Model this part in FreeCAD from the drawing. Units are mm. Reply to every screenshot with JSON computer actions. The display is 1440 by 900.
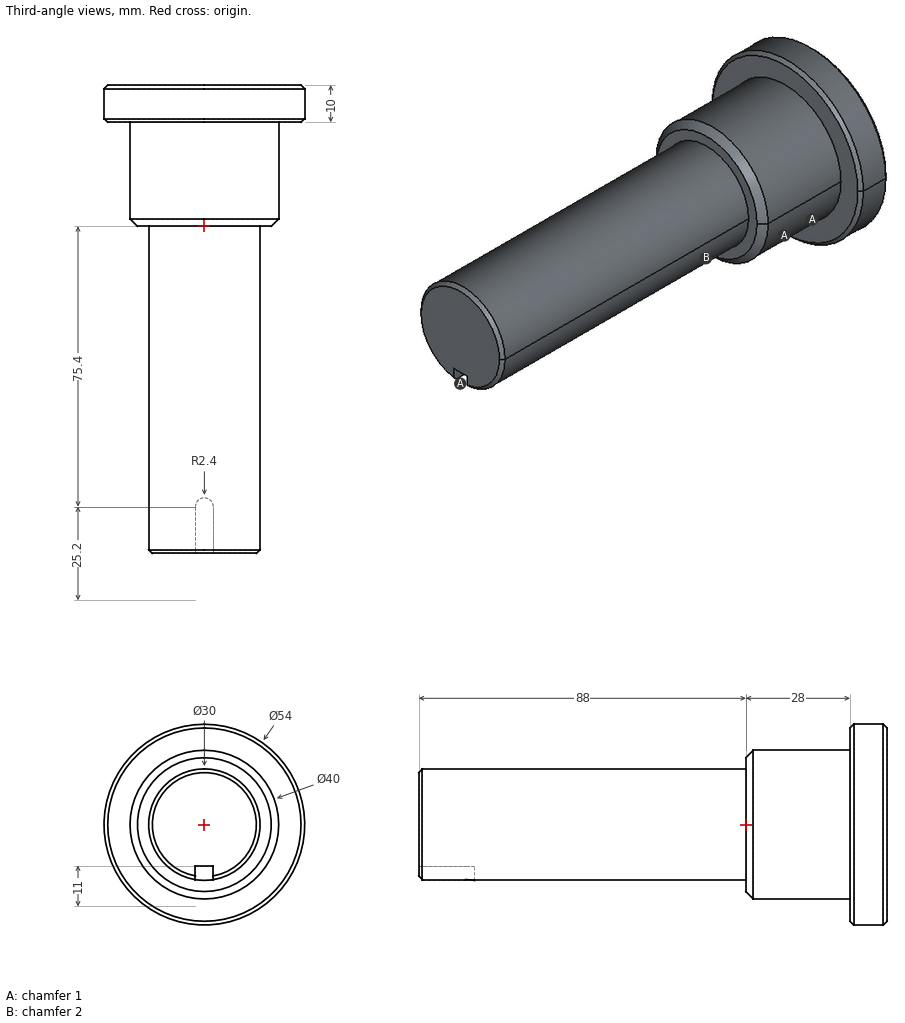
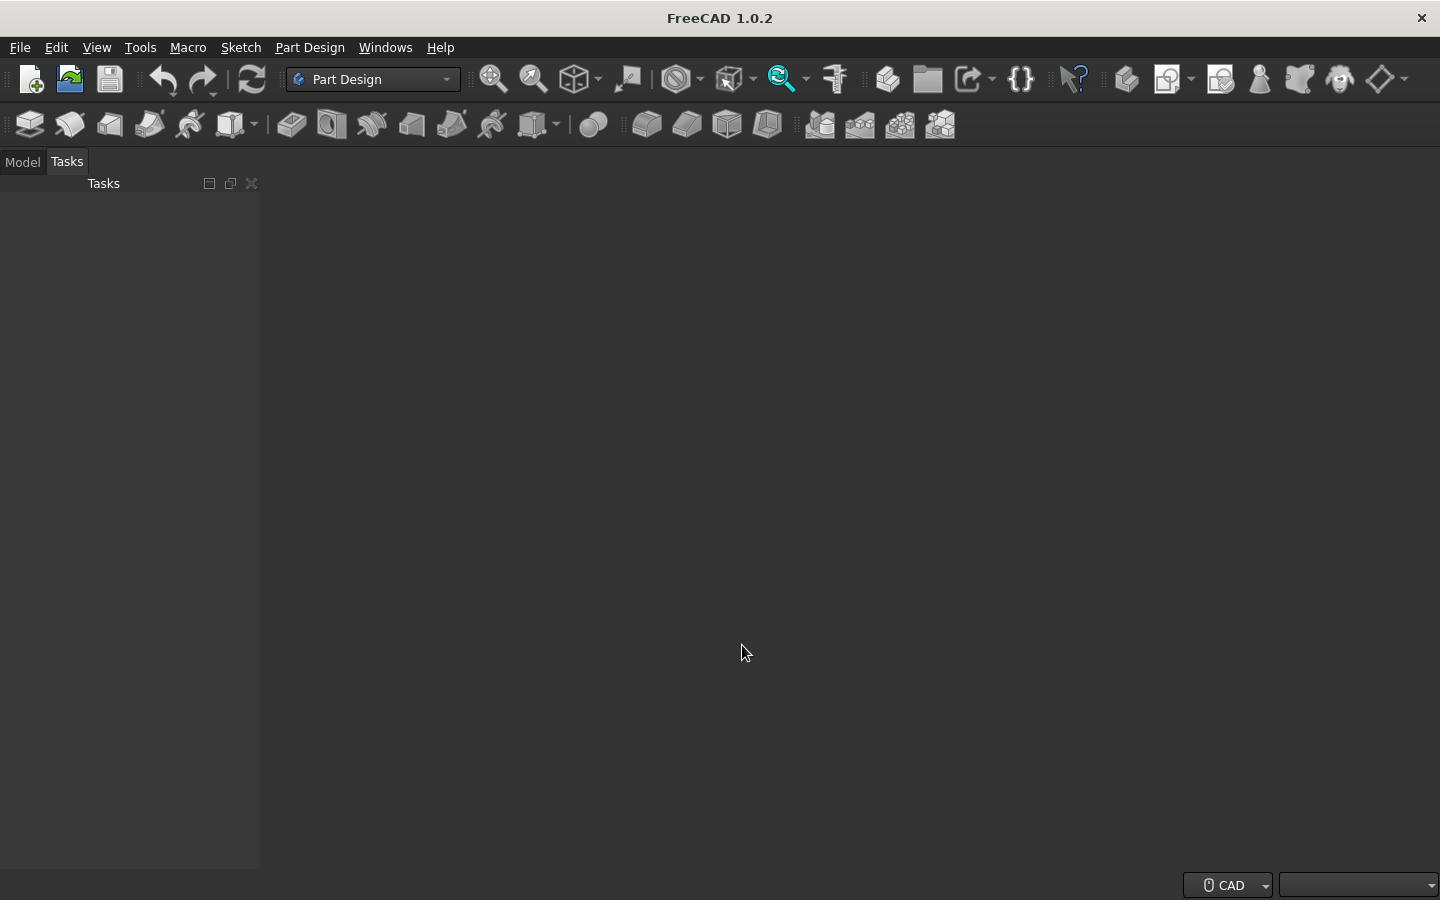
{"action": "left_click", "coordinate": [30, 80]}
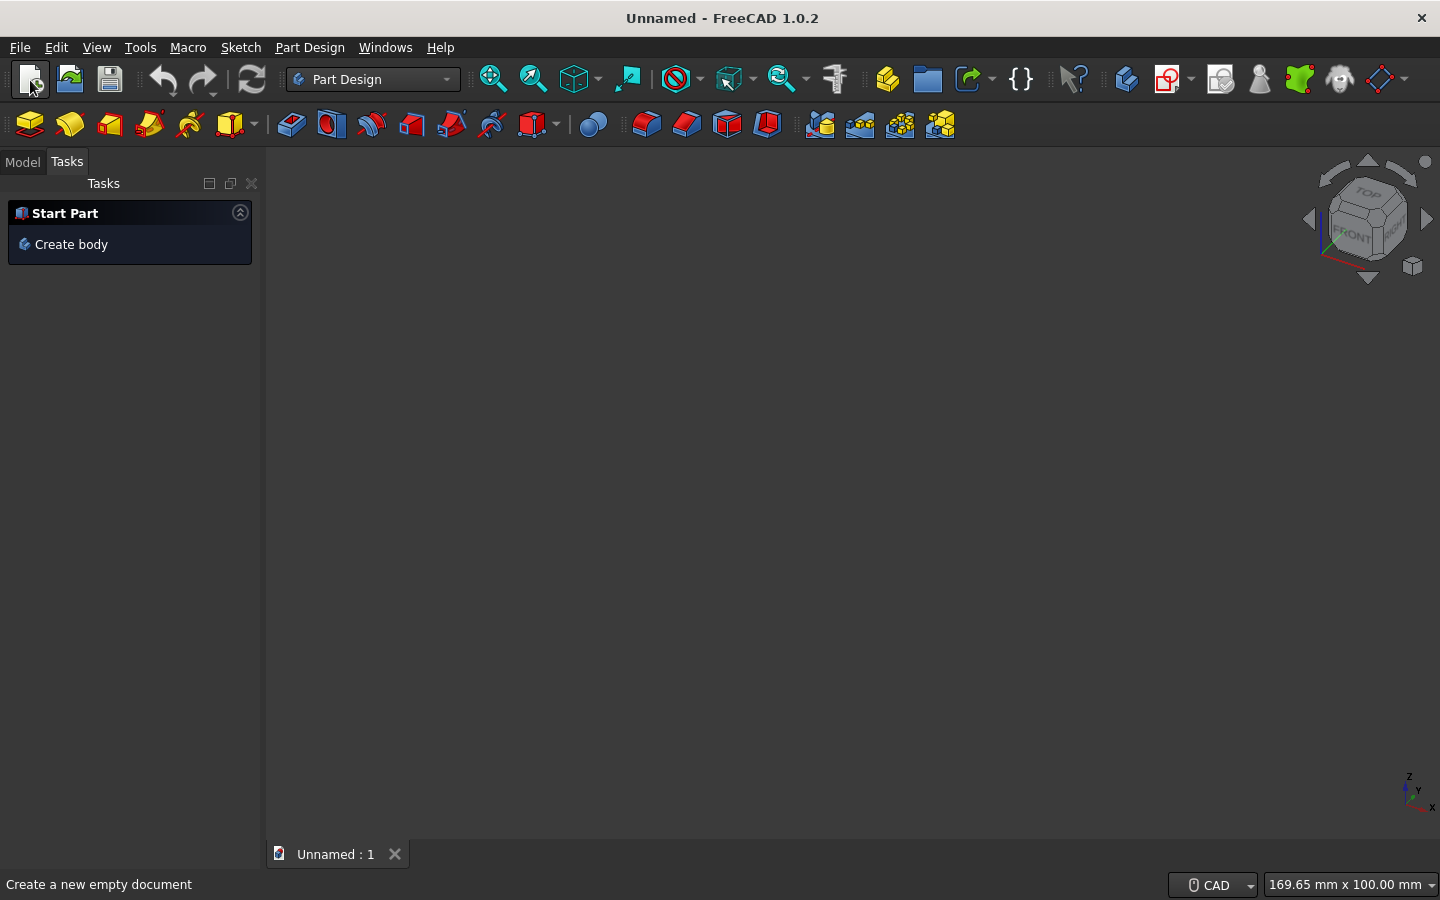
{"action": "left_click", "coordinate": [1168, 80]}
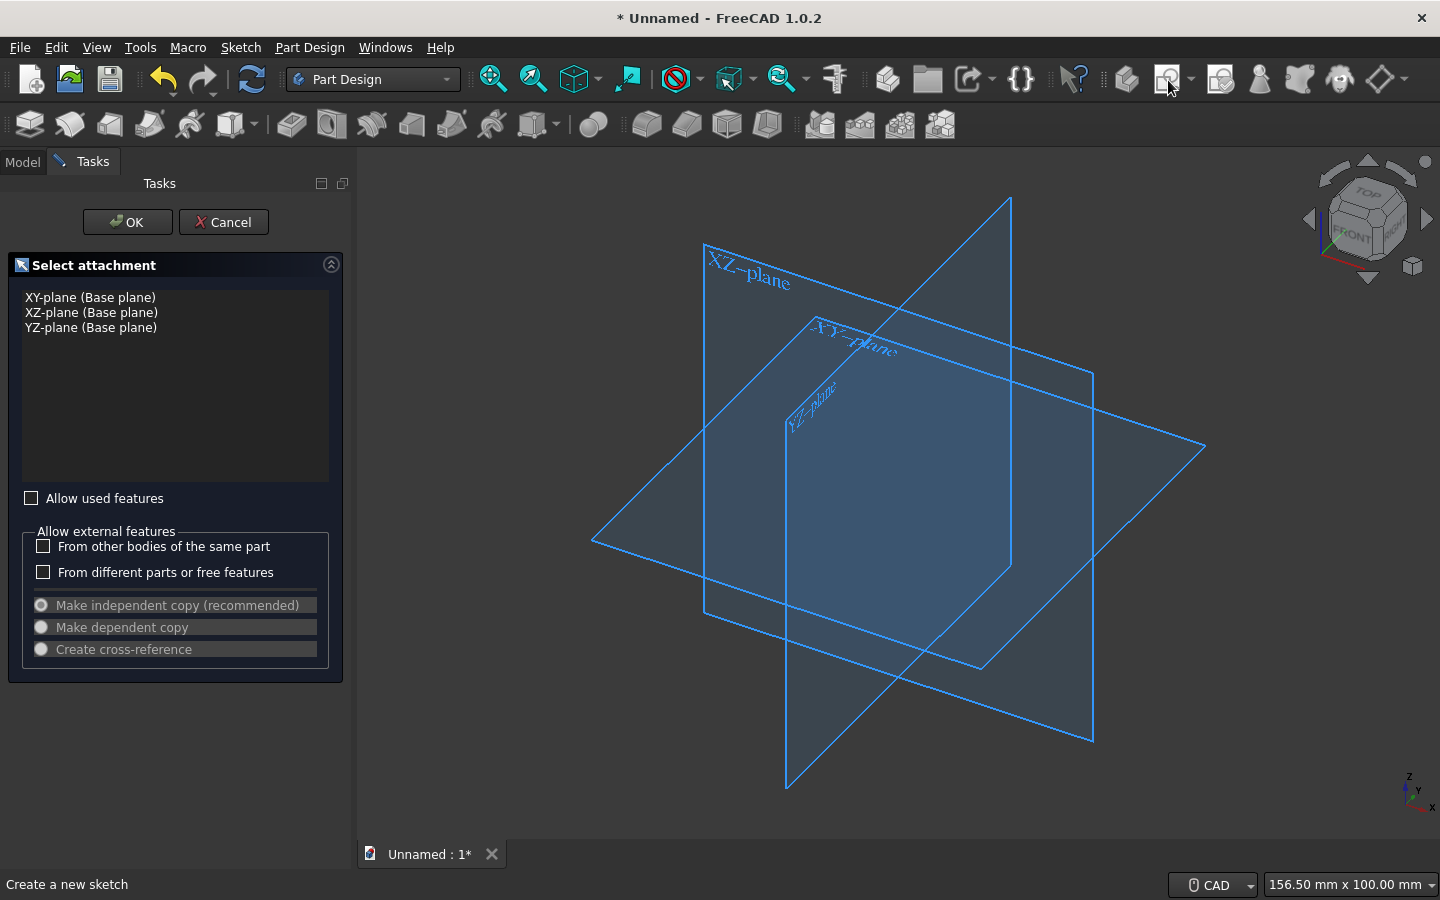
{"action": "left_click", "coordinate": [82, 312]}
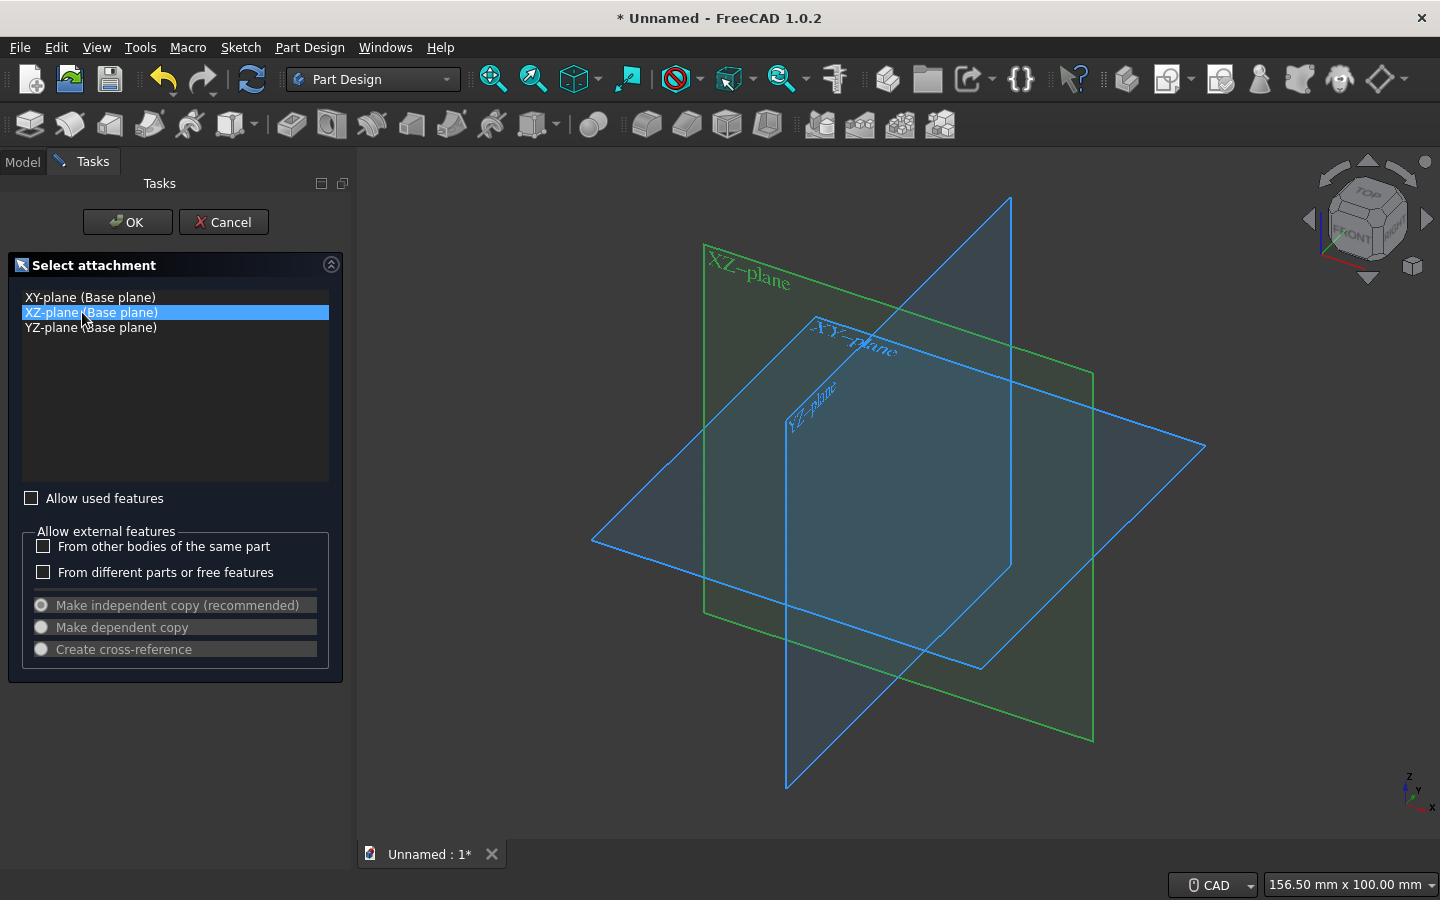
{"action": "left_click", "coordinate": [128, 222]}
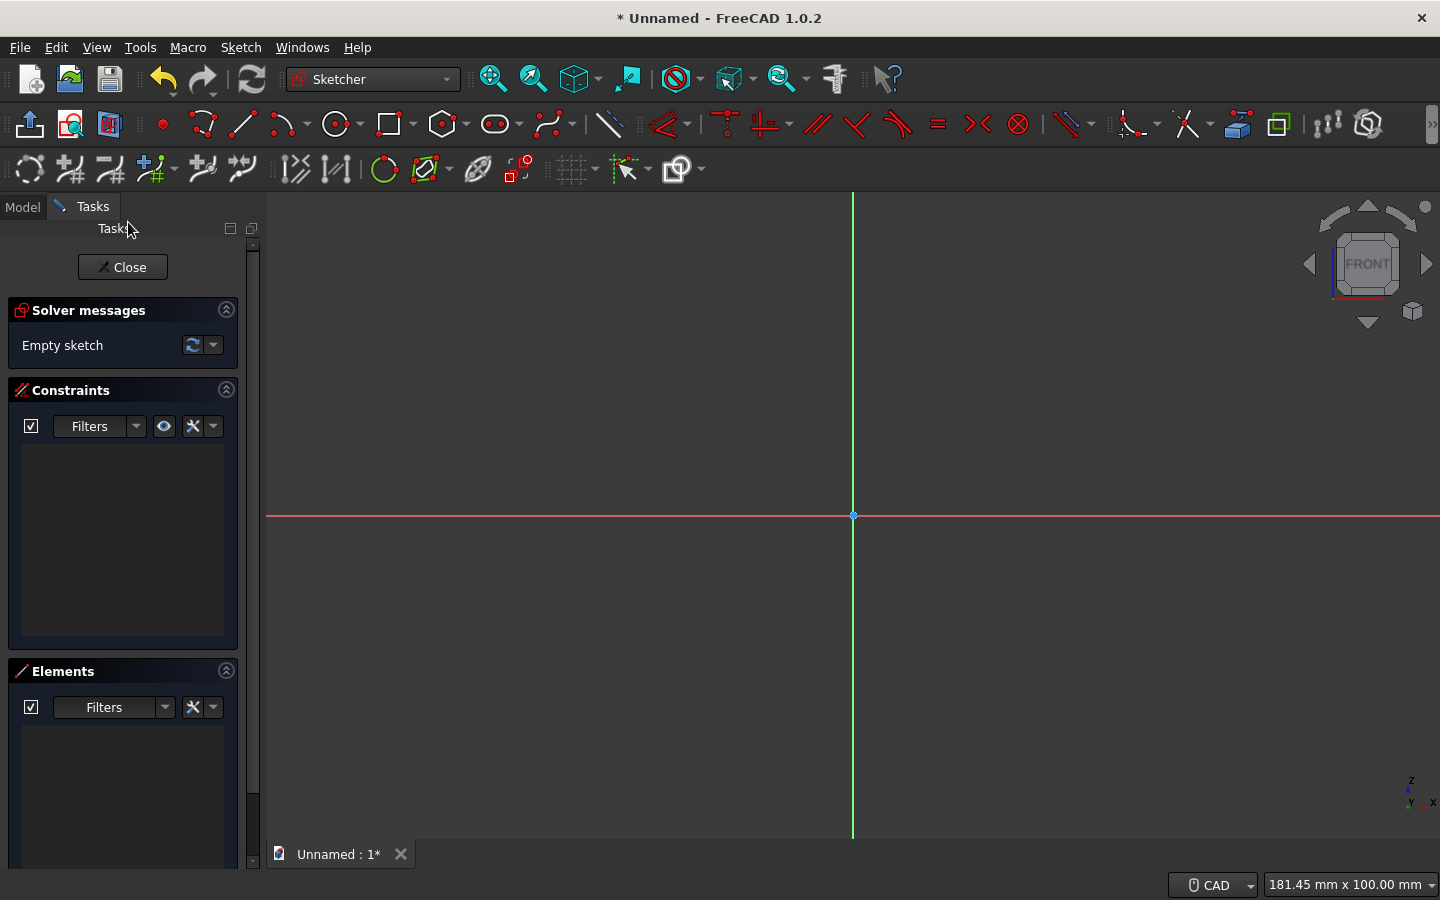
{"action": "scroll", "coordinate": [992, 516], "scroll_direction": "up", "scroll_amount": 2}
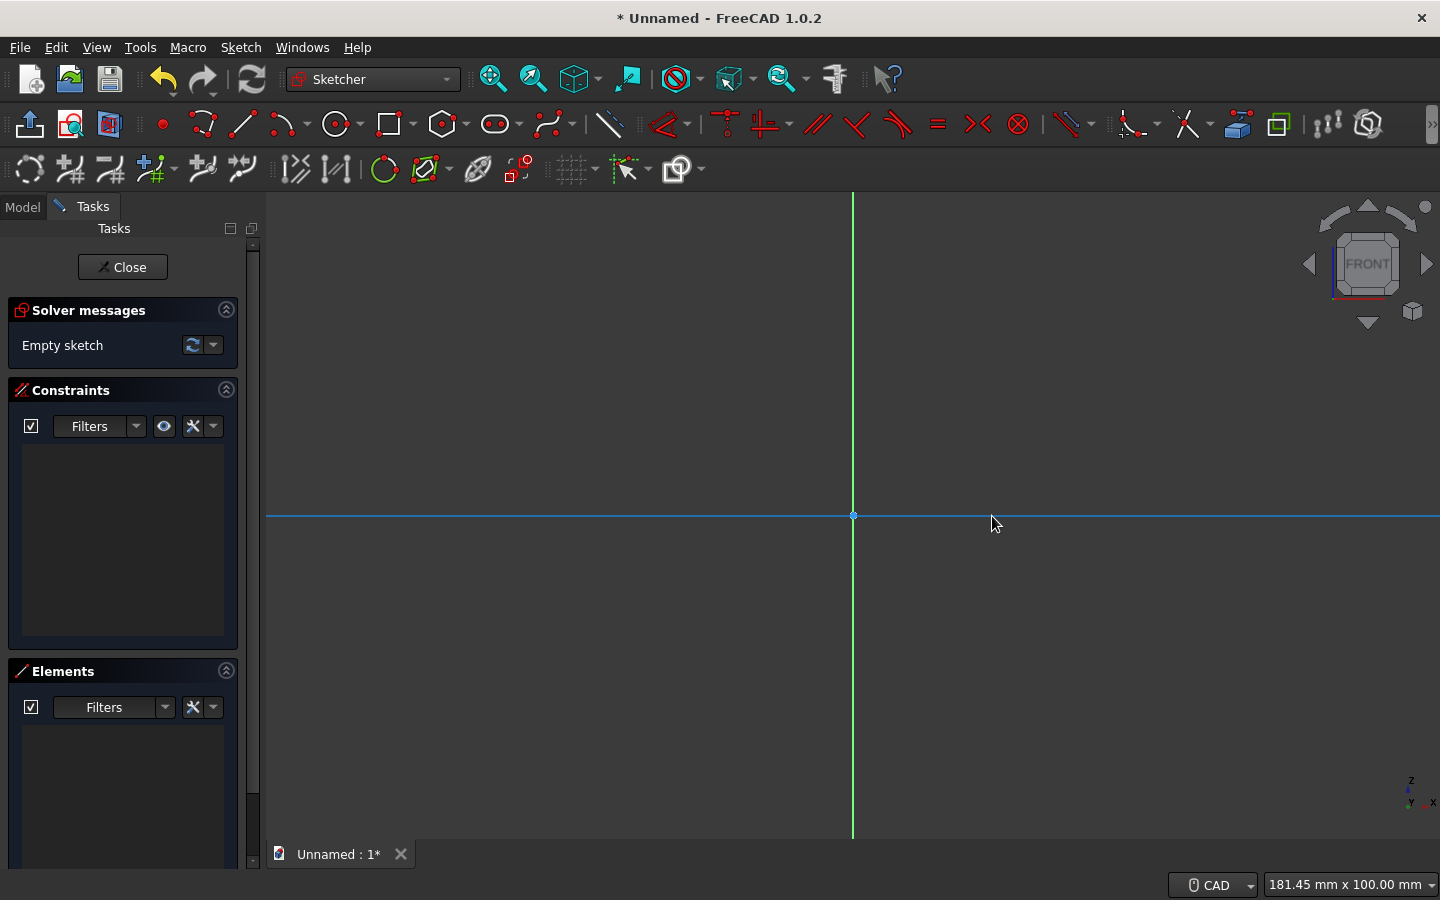
{"action": "key", "text": "g c"}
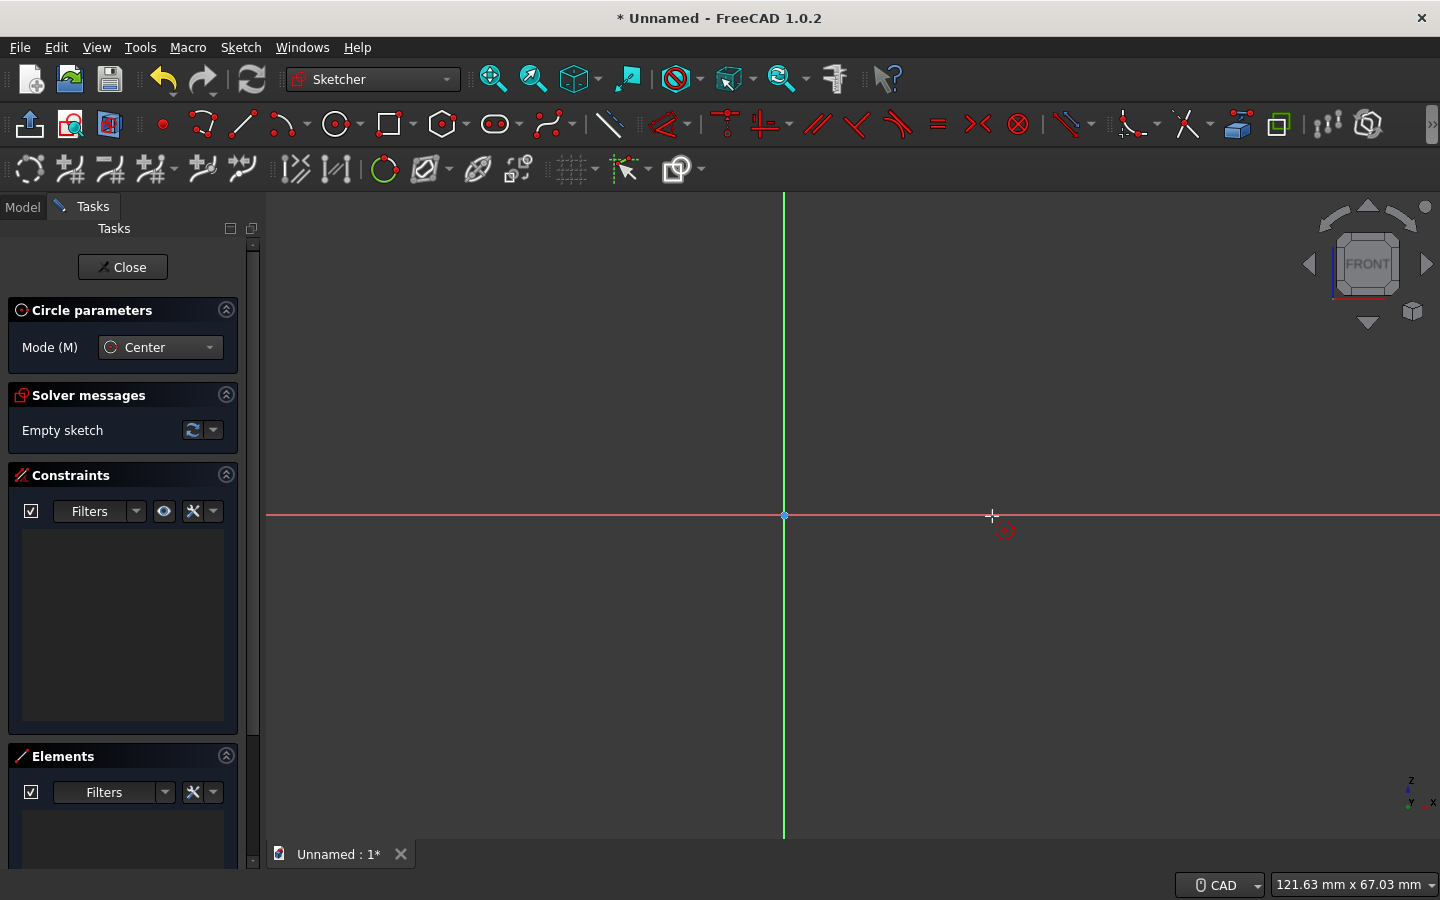
{"action": "left_click", "coordinate": [784, 515]}
{"action": "mouse_move", "coordinate": [921, 379]}